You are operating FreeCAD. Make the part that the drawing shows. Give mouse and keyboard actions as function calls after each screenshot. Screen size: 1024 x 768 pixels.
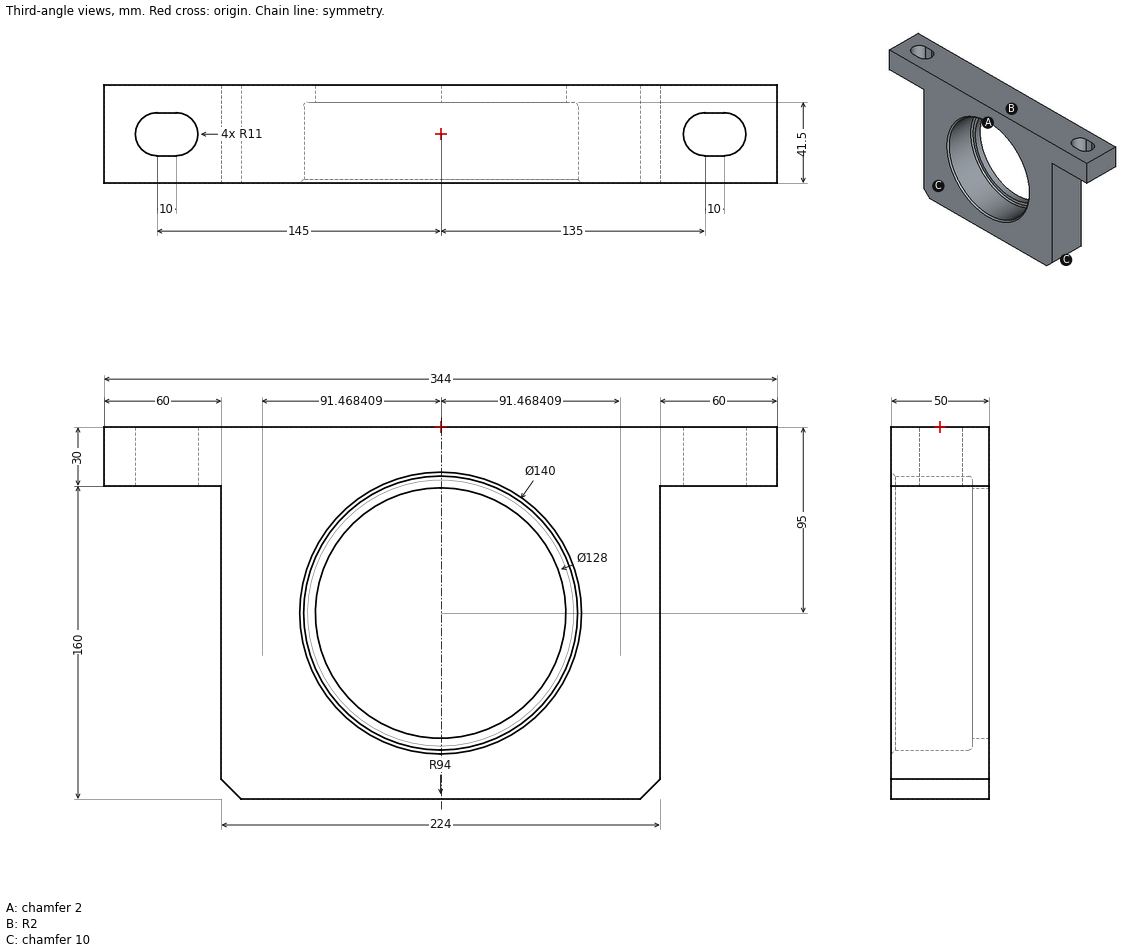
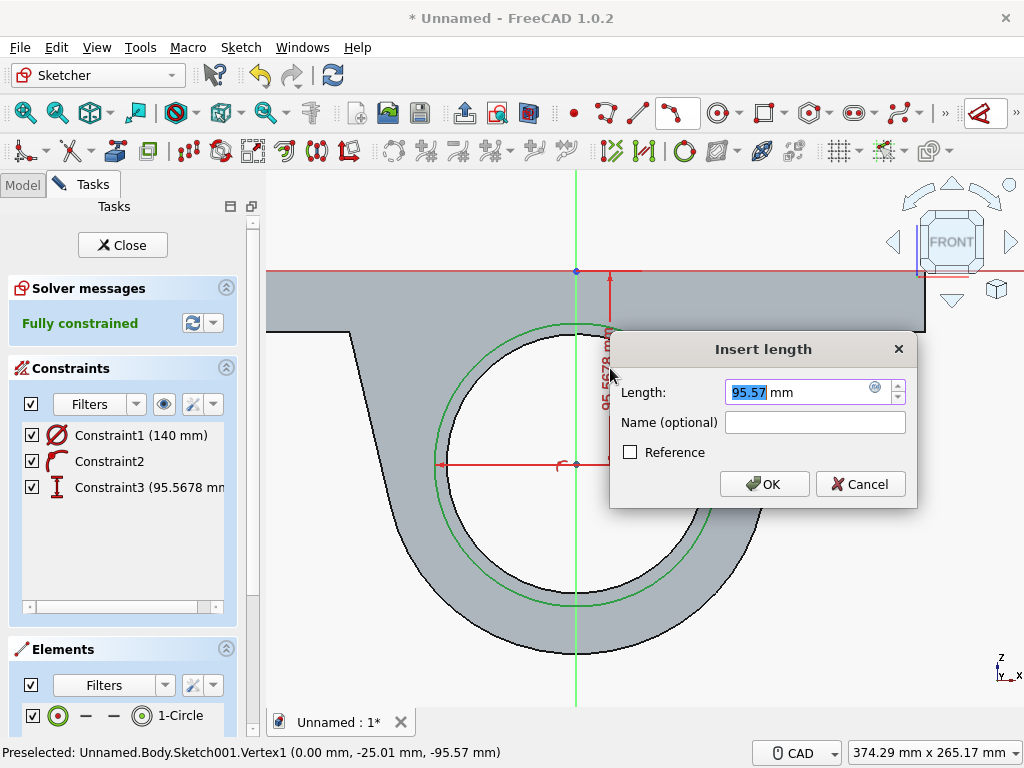
text(95)
key(Return)
key(Escape)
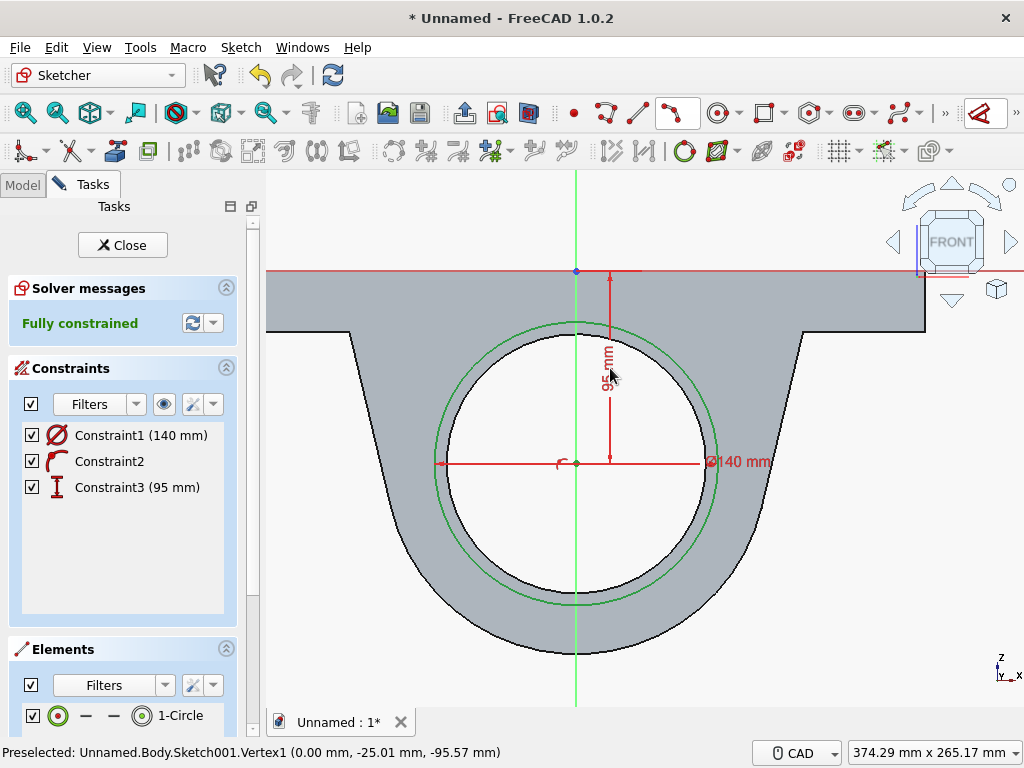
click(123, 245)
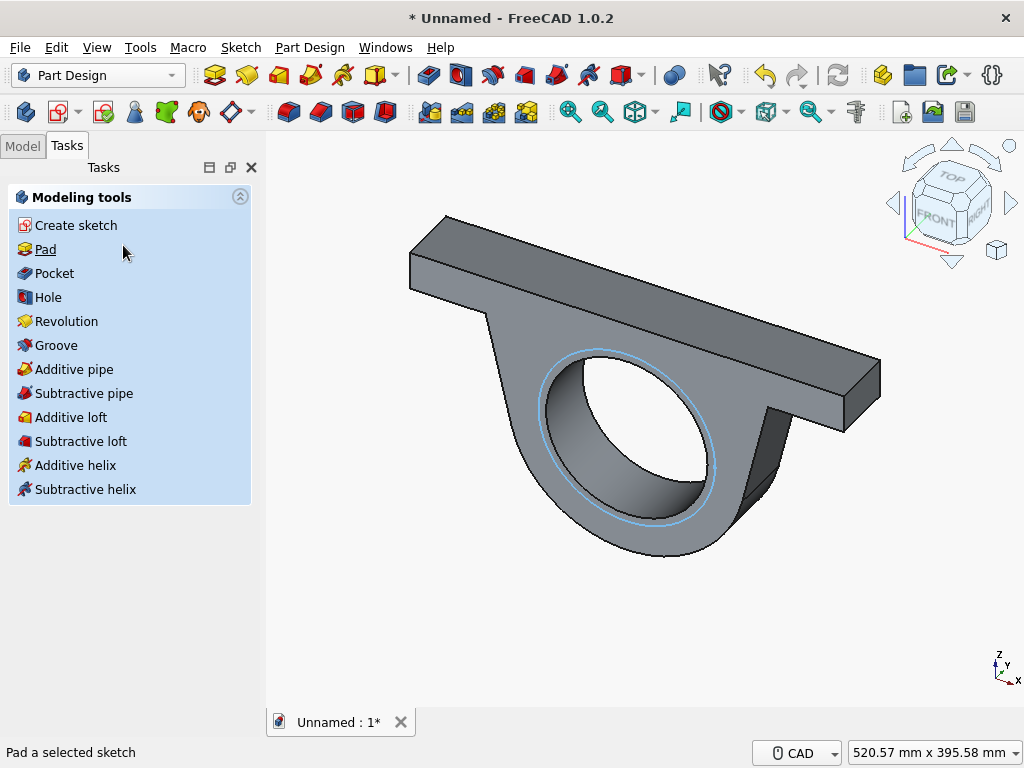
click(430, 76)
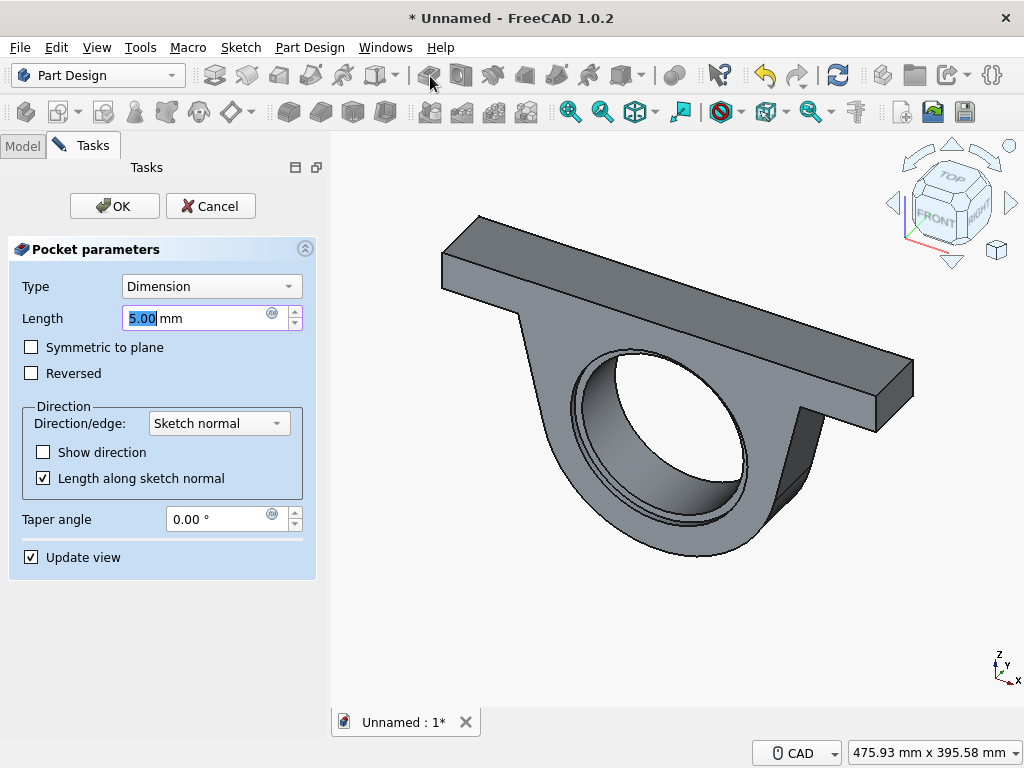
text(41.5)
key(Tab)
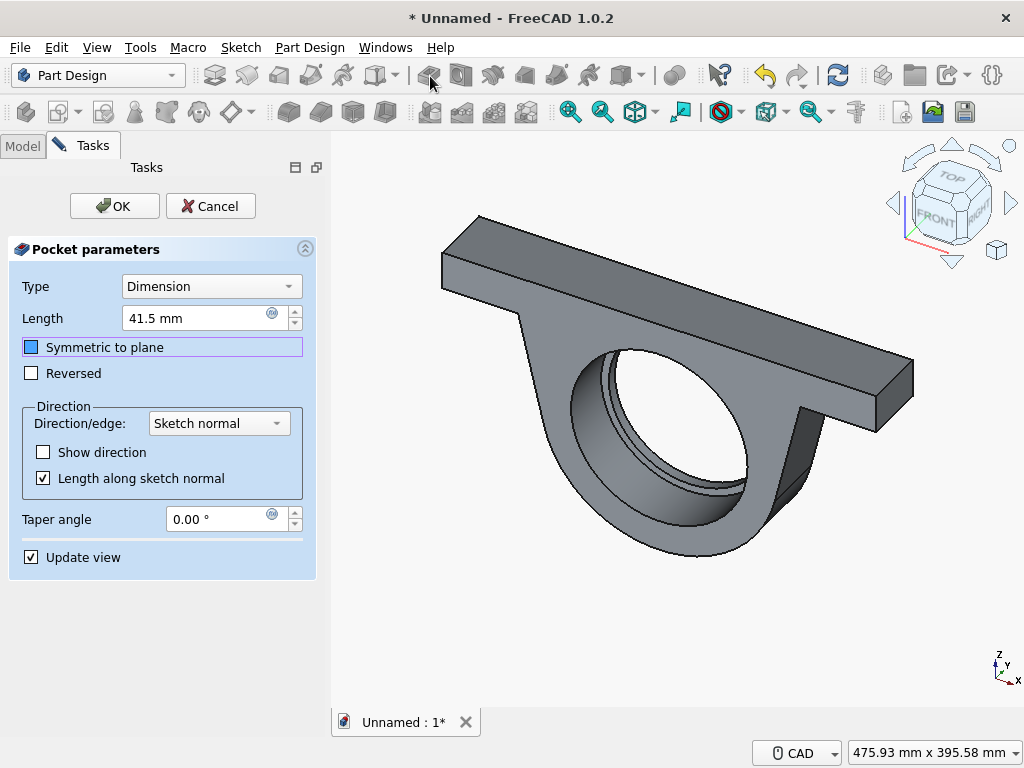
click(115, 206)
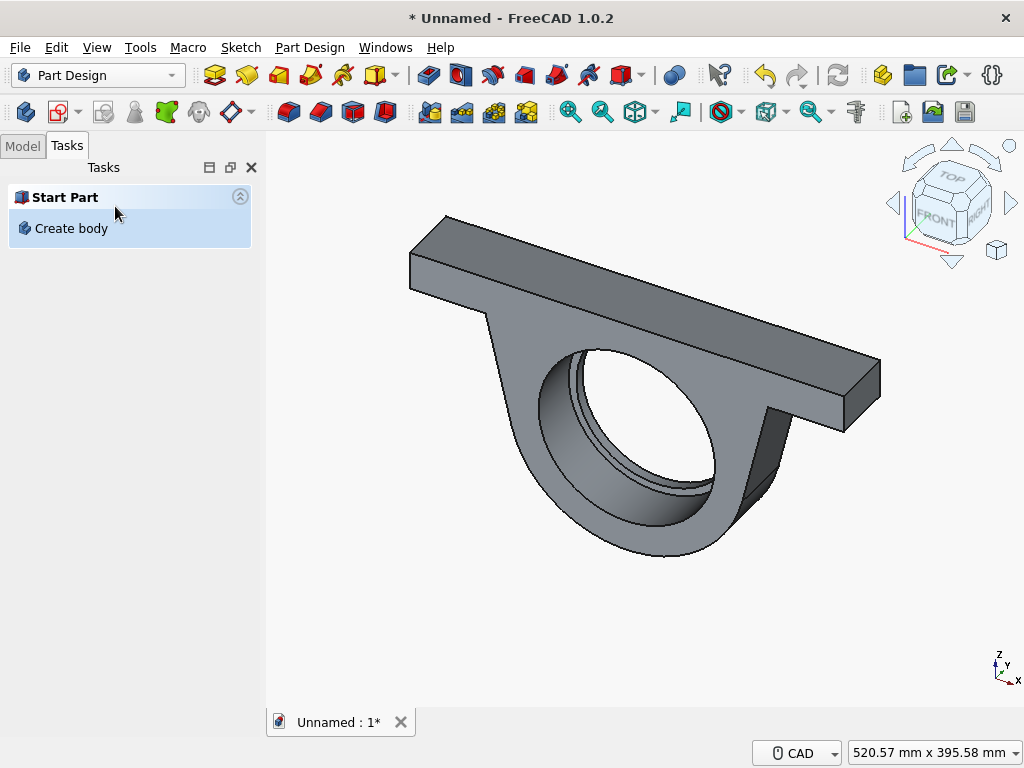
click(539, 408)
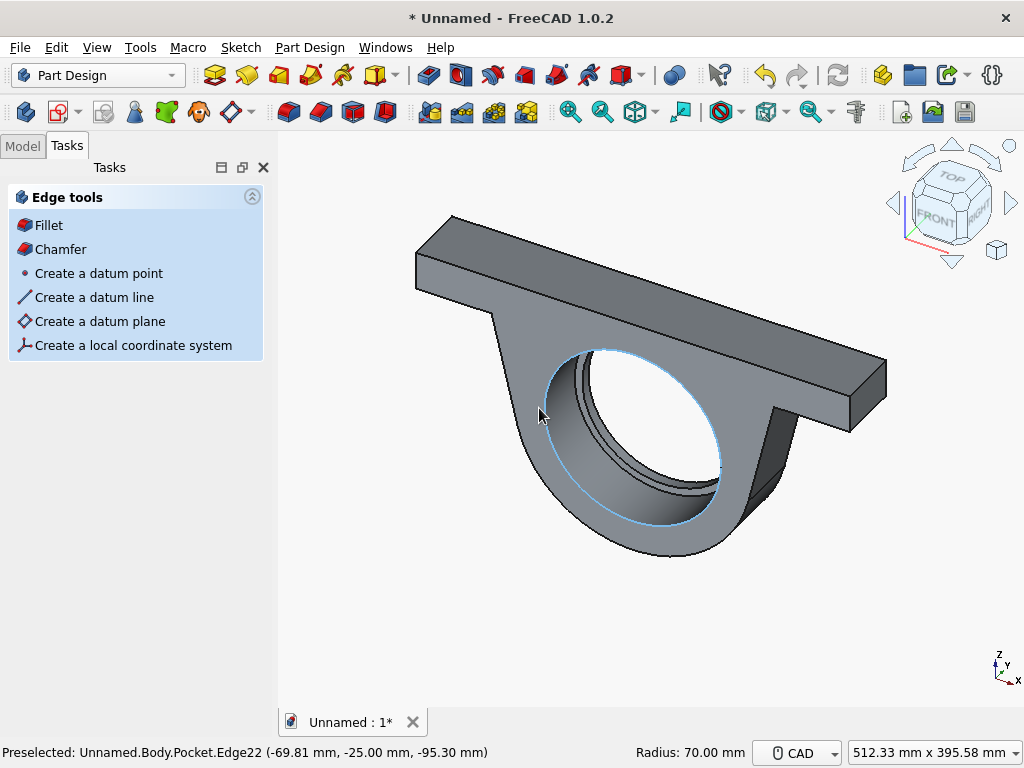
click(322, 112)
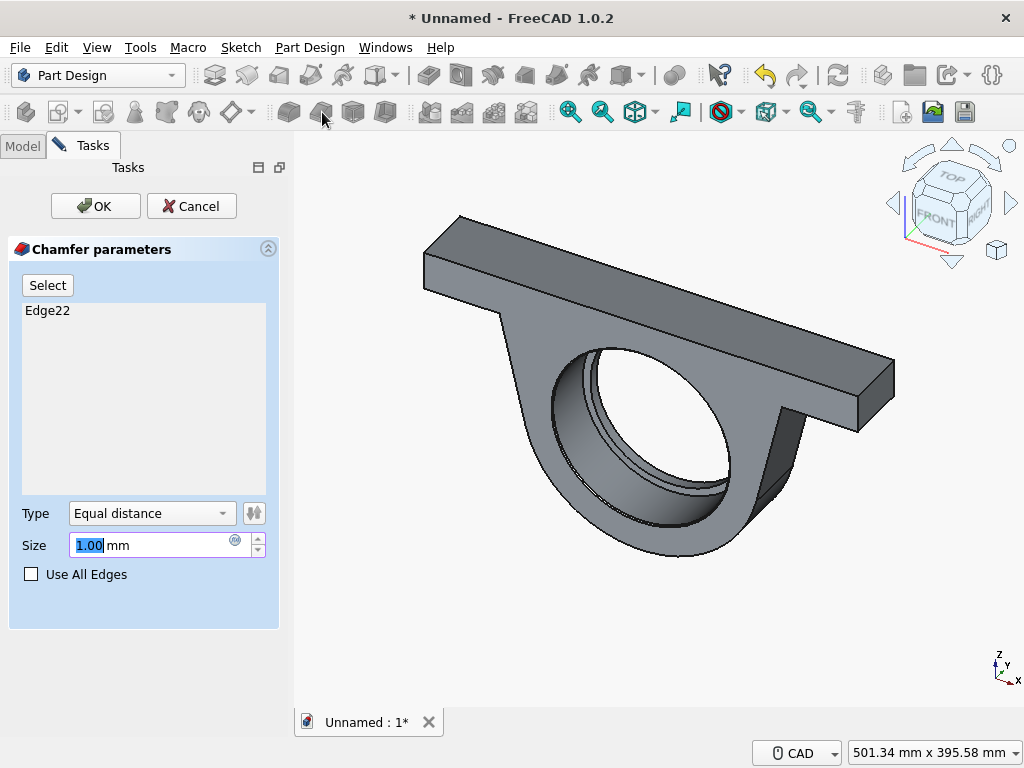
text(2)
key(Tab)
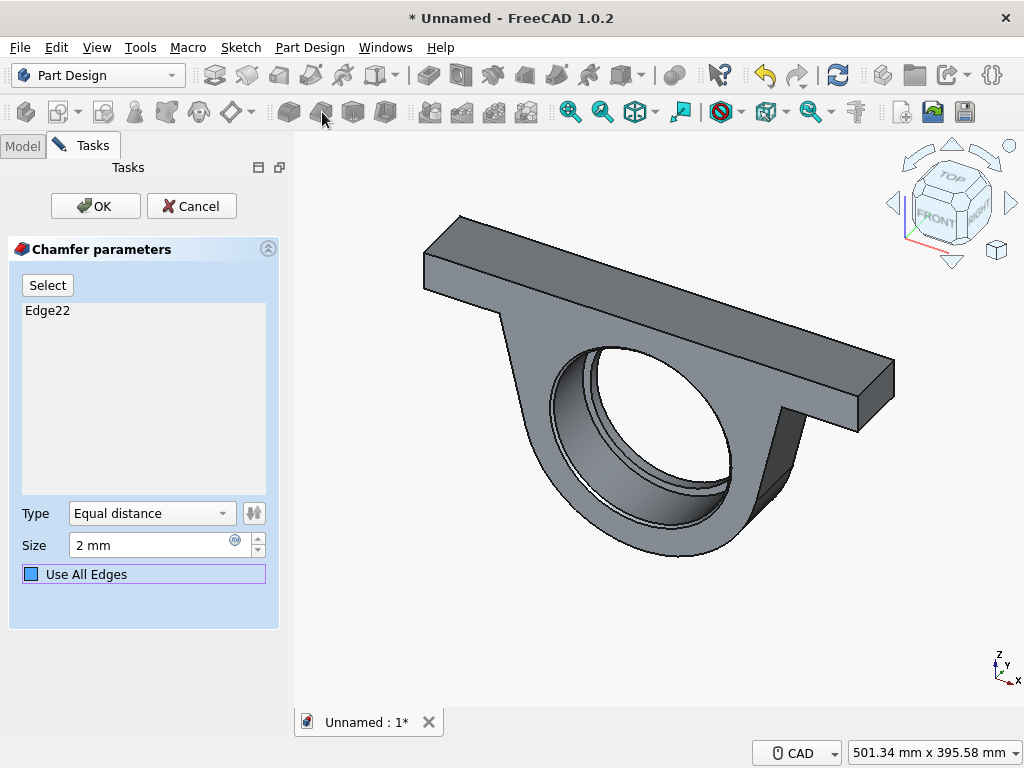
click(96, 206)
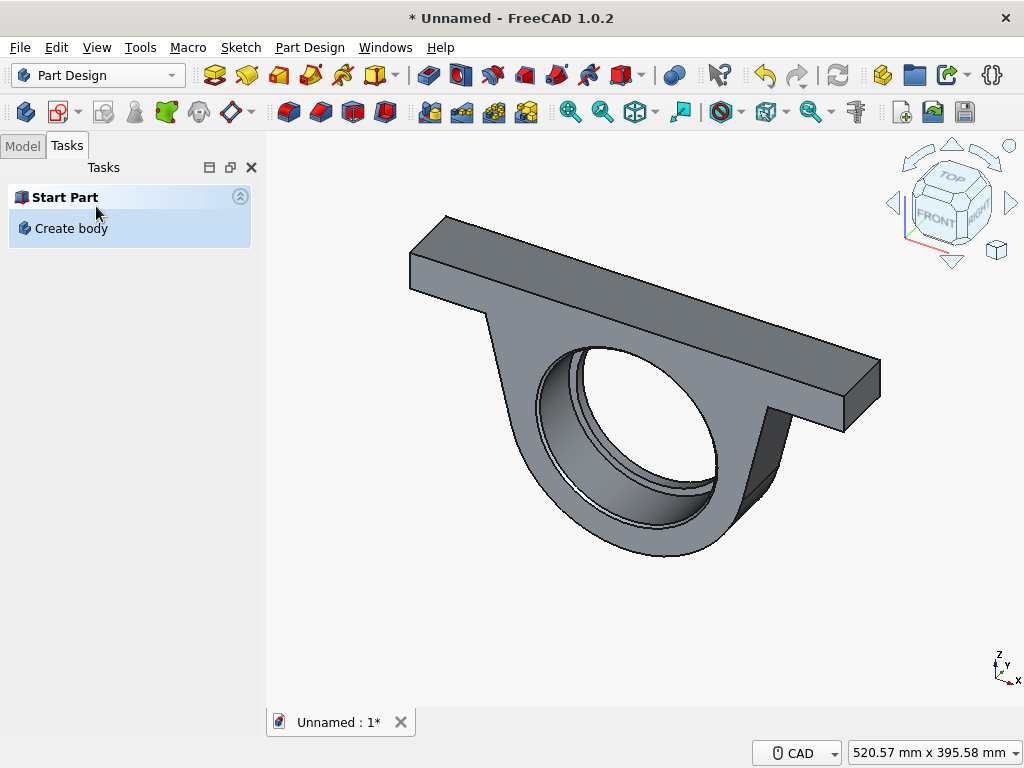
key(0)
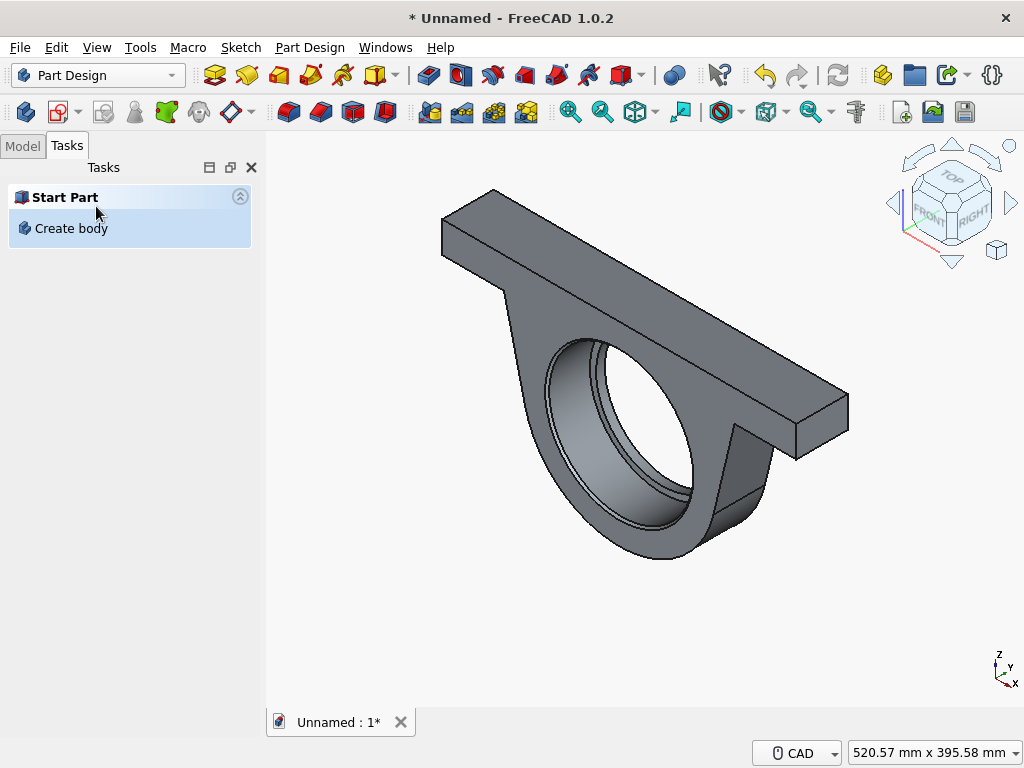
key(2)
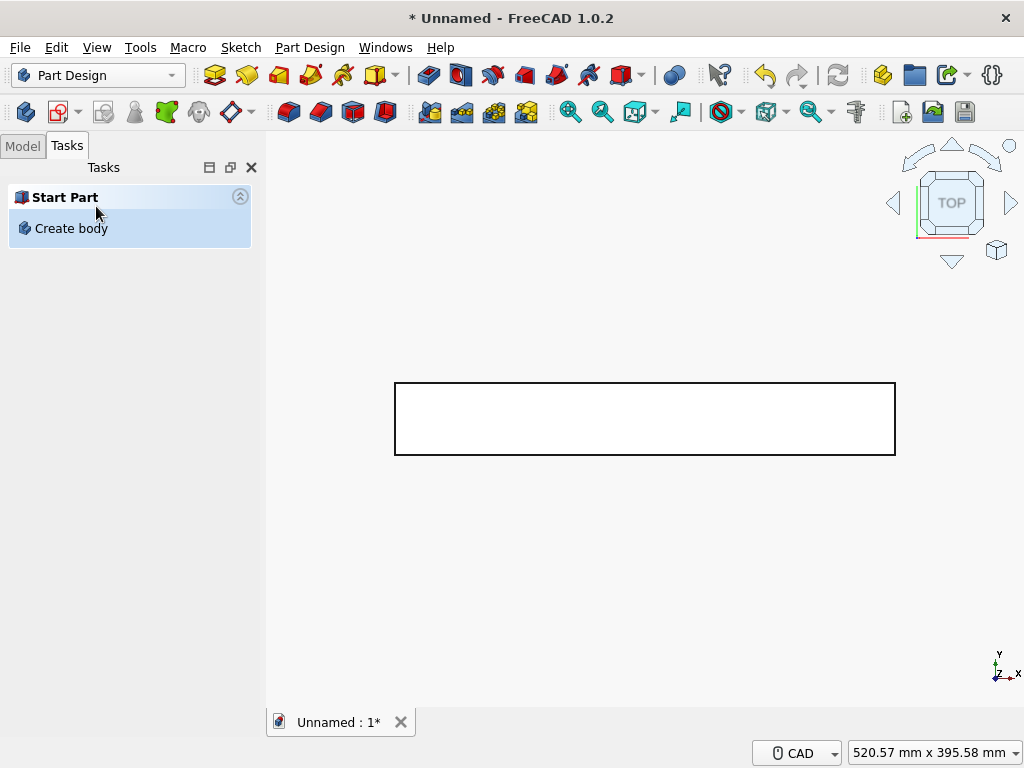
key(1)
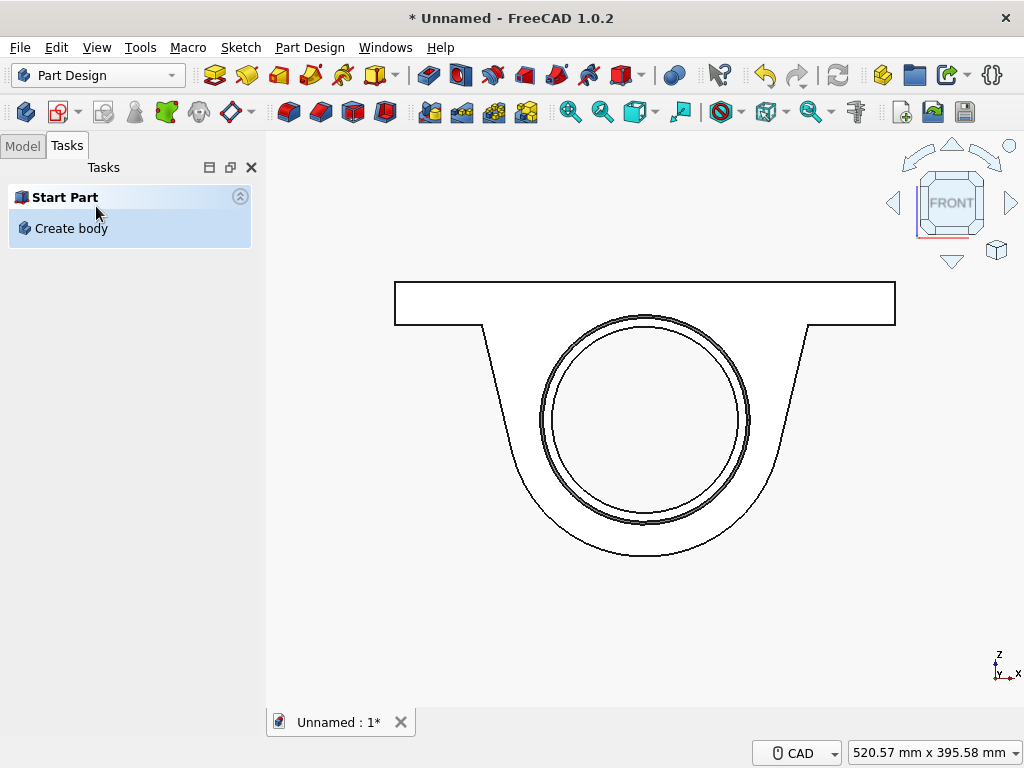
key(3)